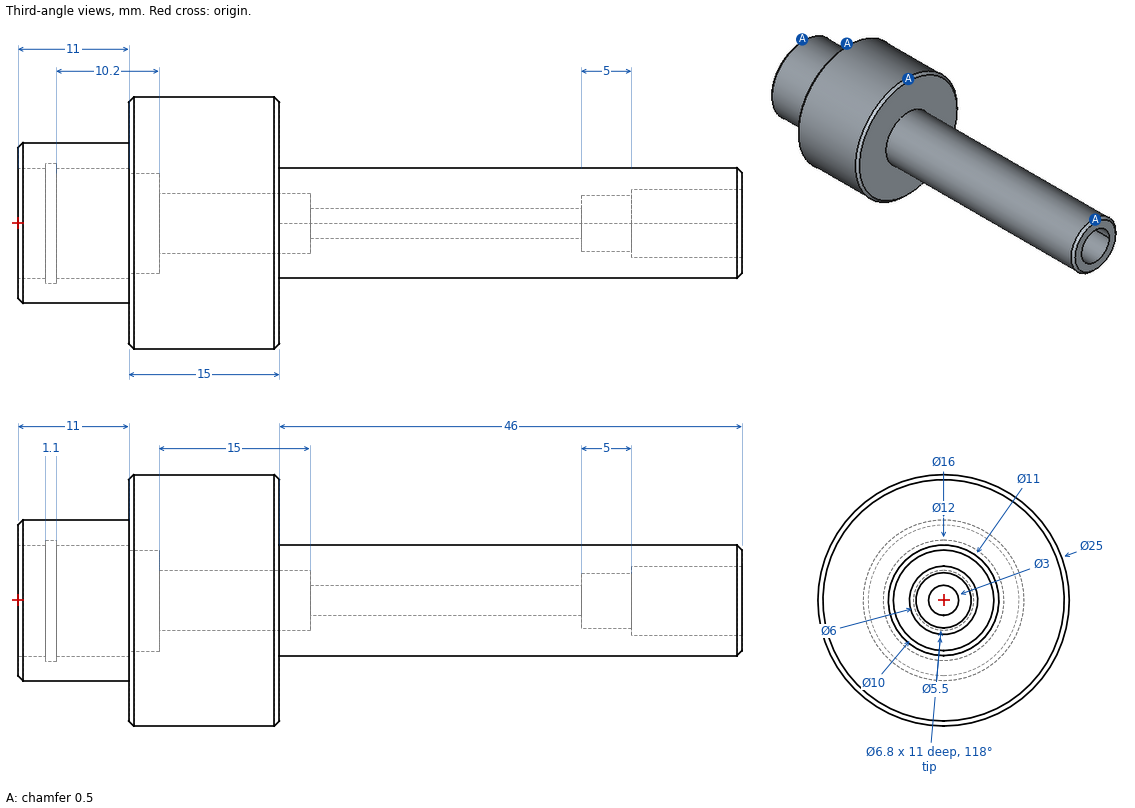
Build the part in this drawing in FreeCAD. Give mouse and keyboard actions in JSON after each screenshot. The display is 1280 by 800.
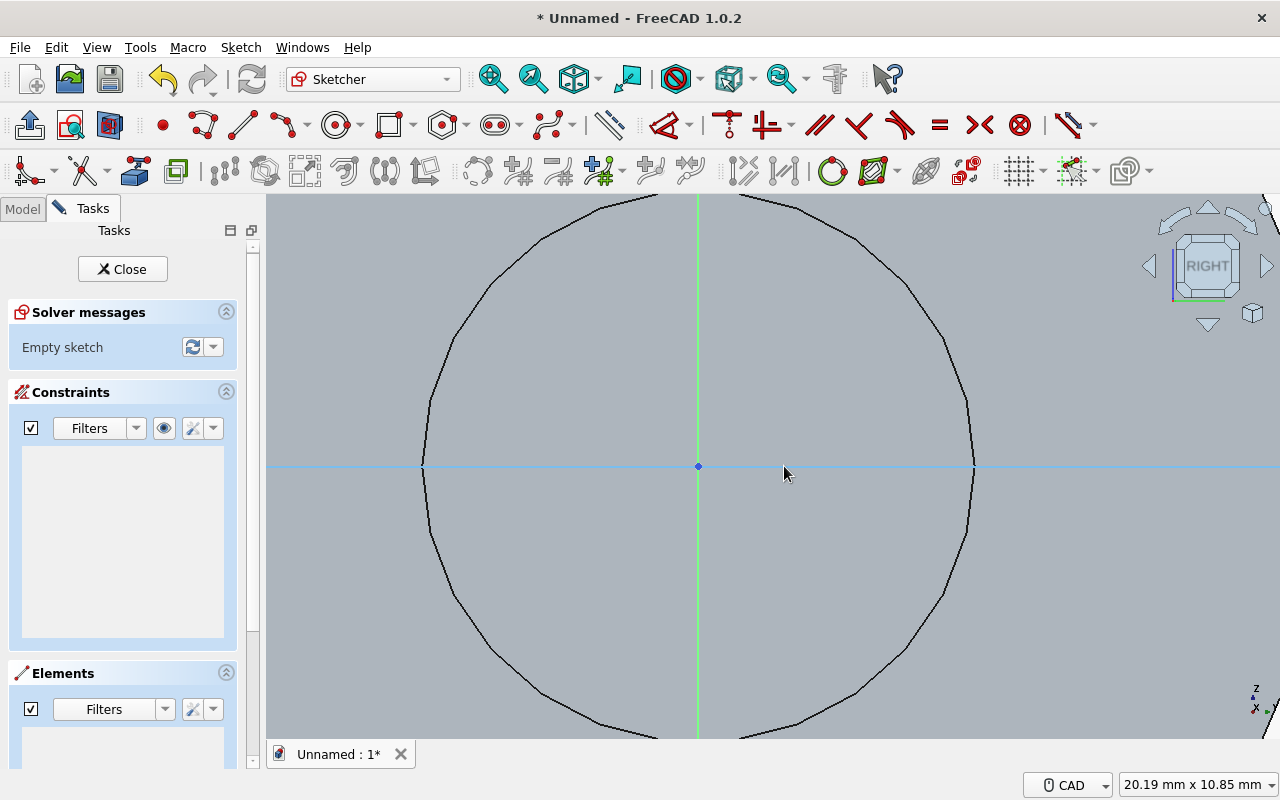
{"action": "left_click", "coordinate": [336, 126]}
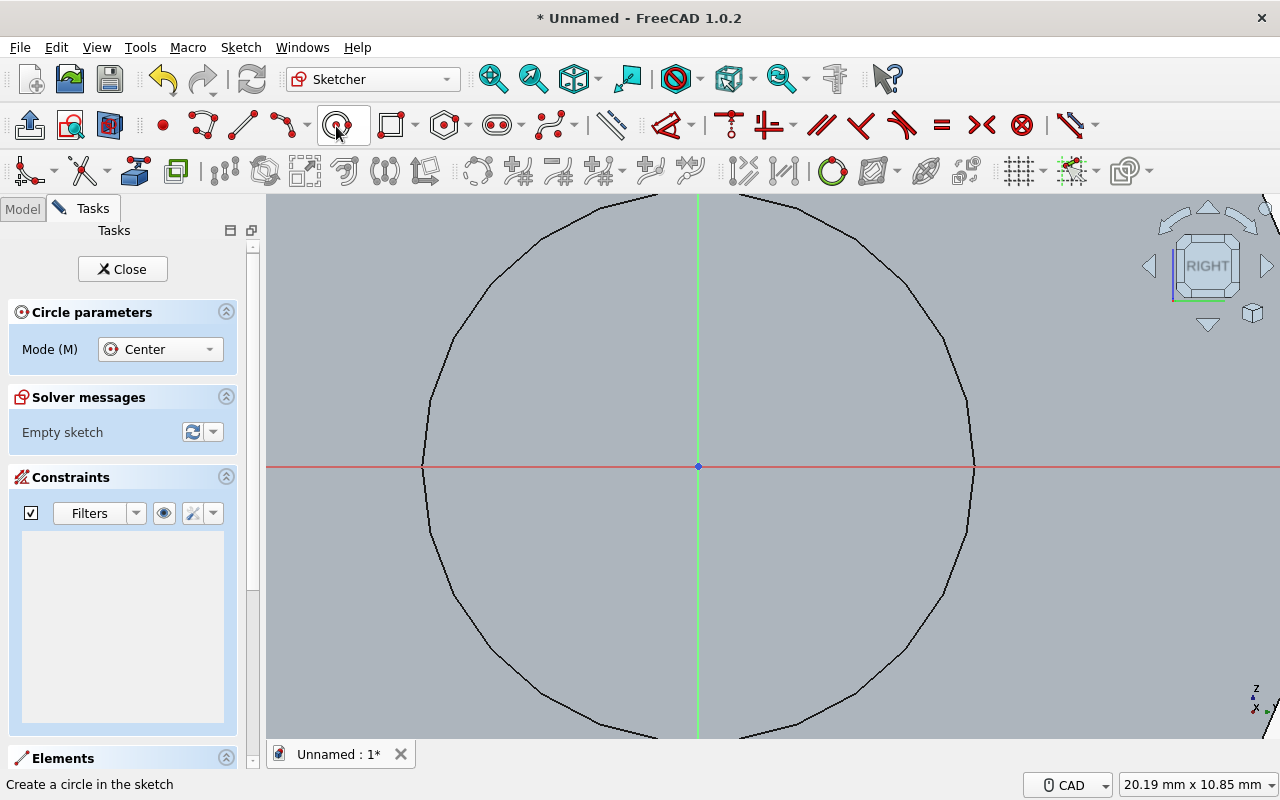
{"action": "left_click", "coordinate": [698, 466]}
{"action": "mouse_move", "coordinate": [819, 346]}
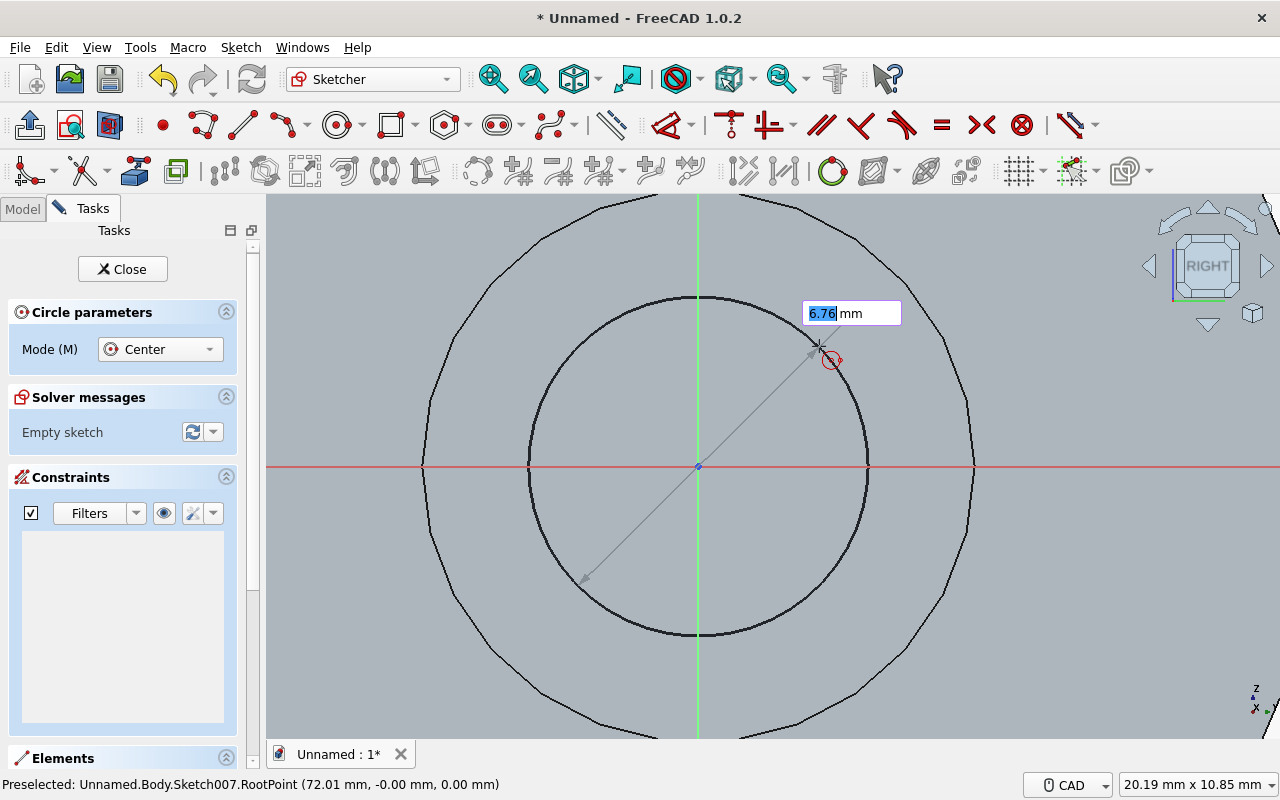
{"action": "type", "text": "6.8"}
{"action": "key", "text": "Return"}
{"action": "key", "text": "Escape"}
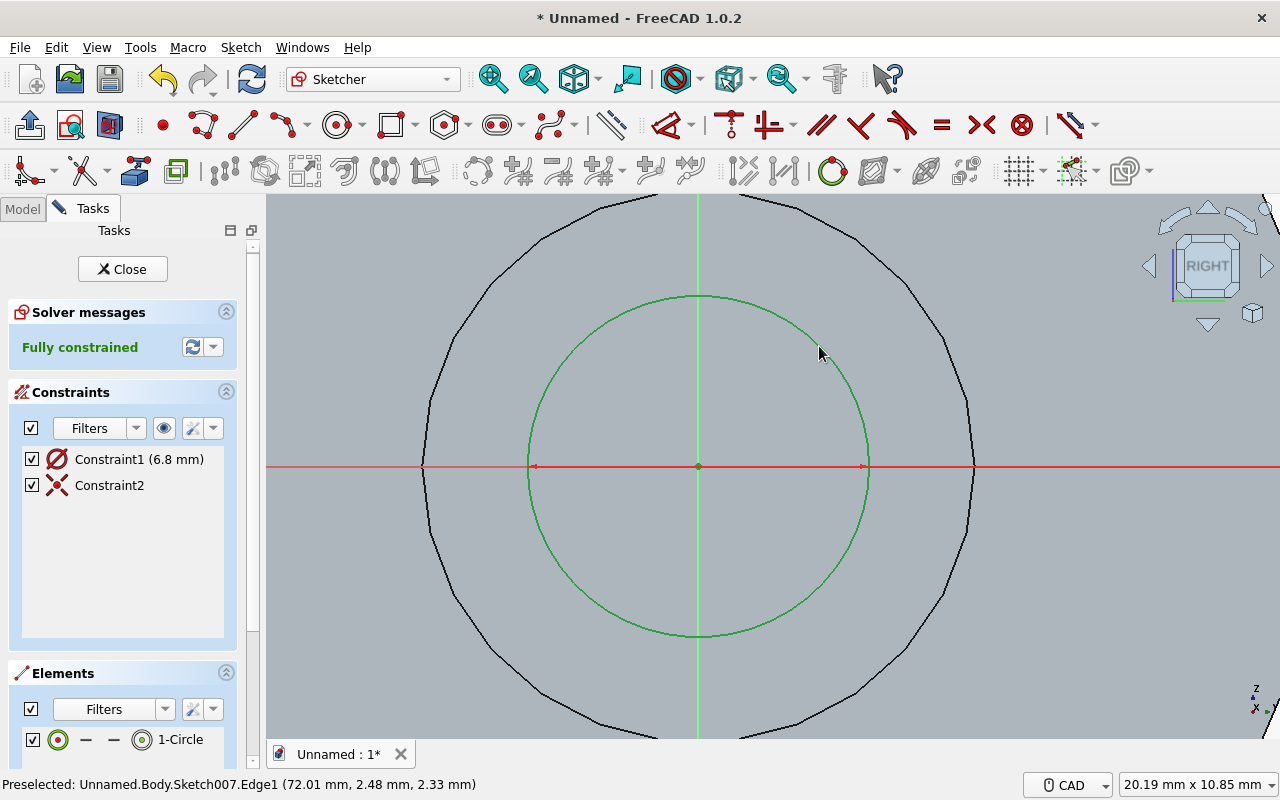
{"action": "left_click", "coordinate": [123, 269]}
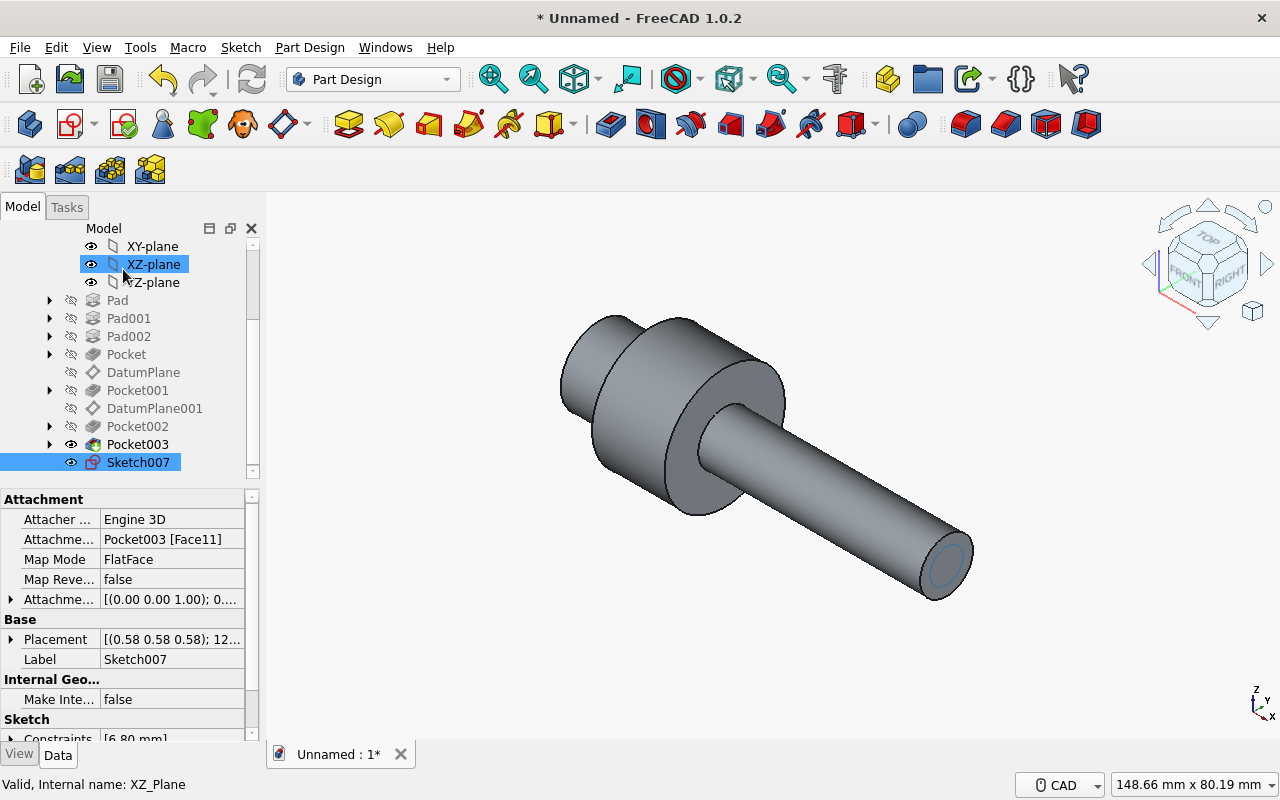
{"action": "left_click", "coordinate": [652, 124]}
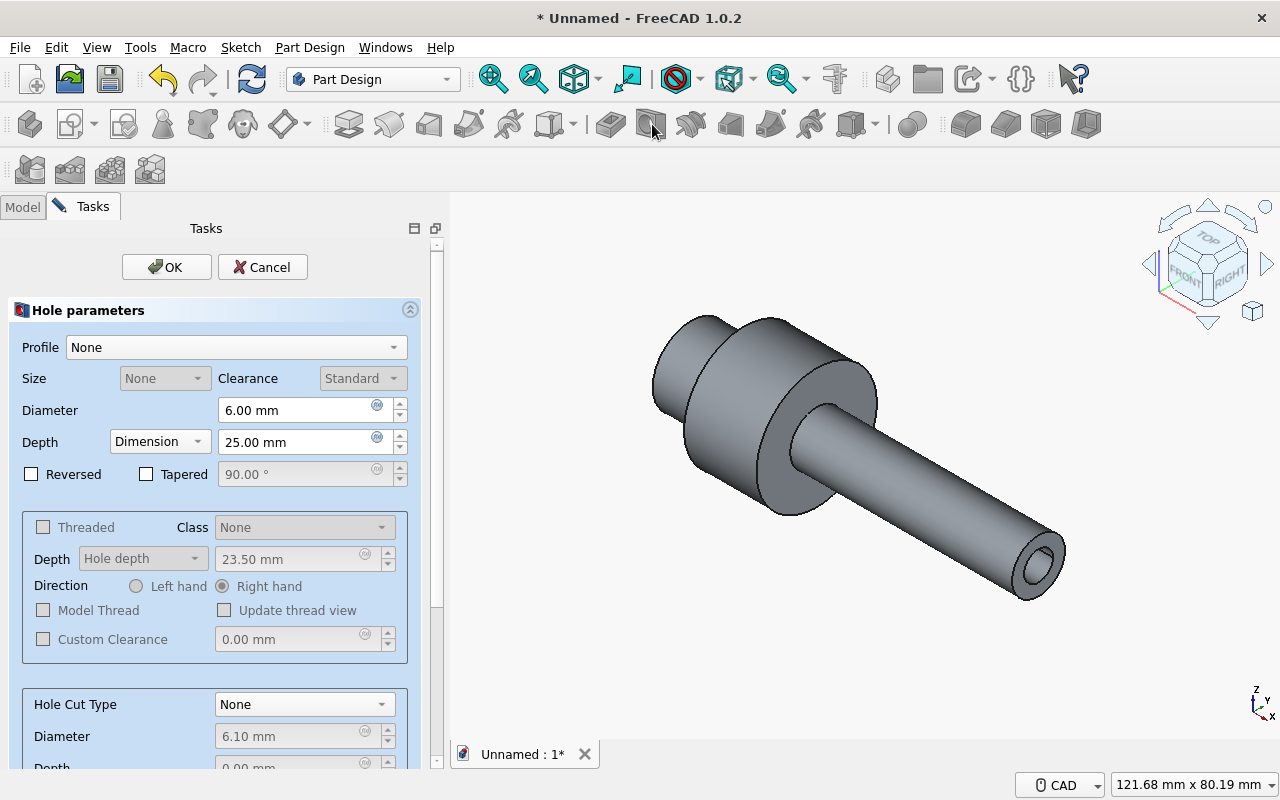
{"action": "triple_click", "coordinate": [305, 410]}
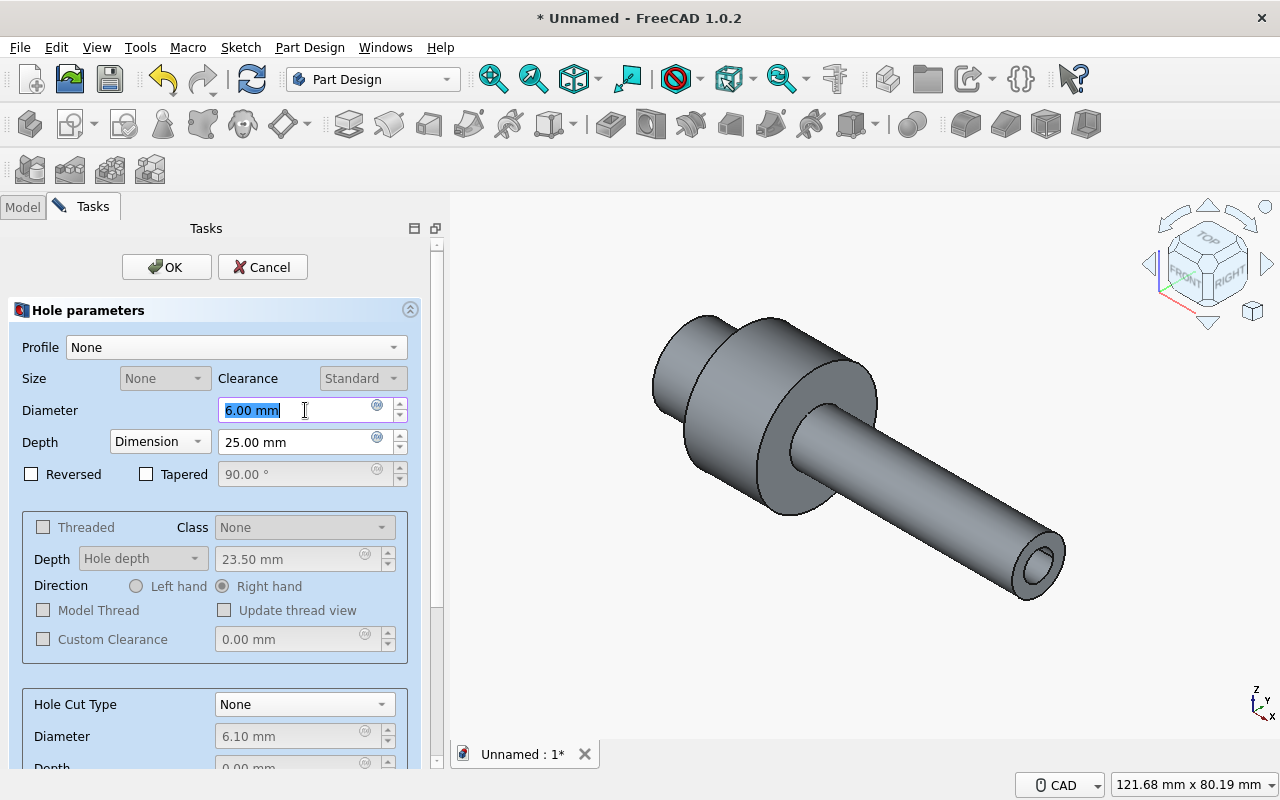
{"action": "type", "text": "6.8"}
{"action": "key", "text": "Tab"}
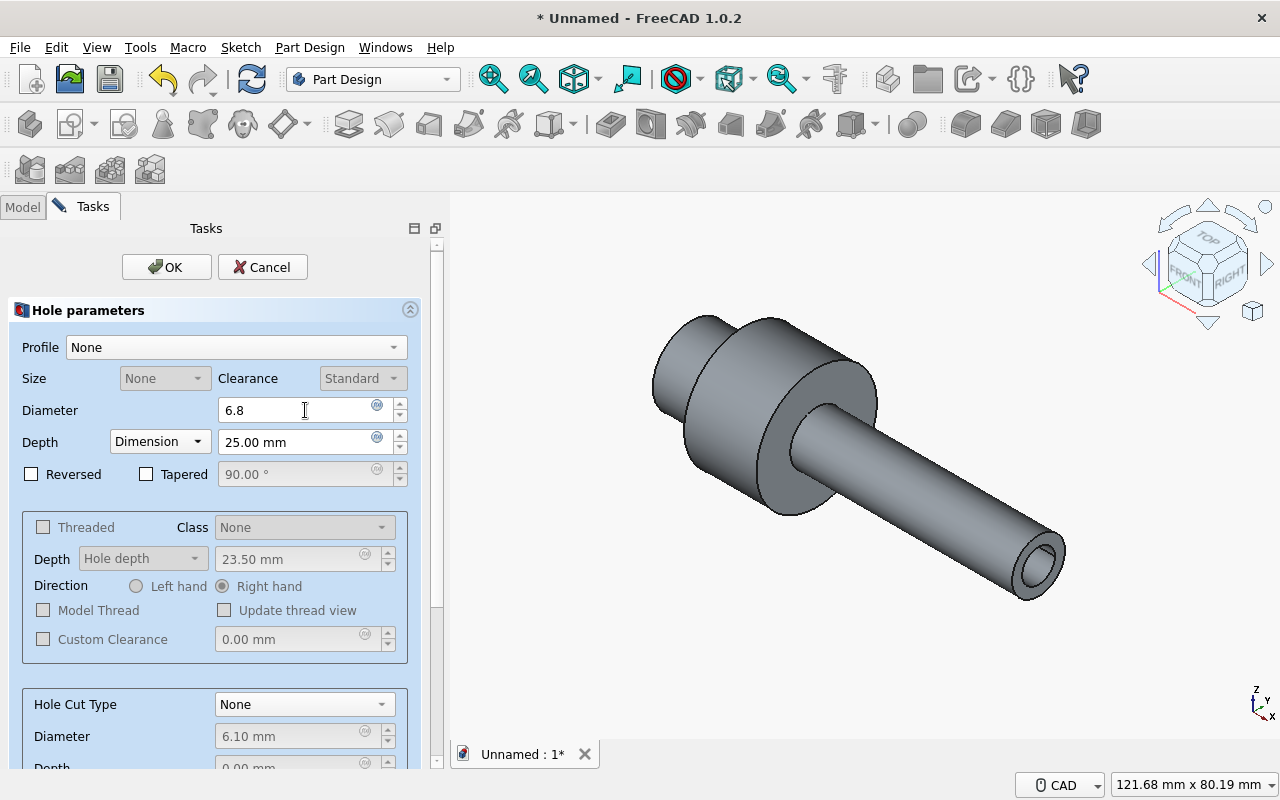
{"action": "triple_click", "coordinate": [305, 442]}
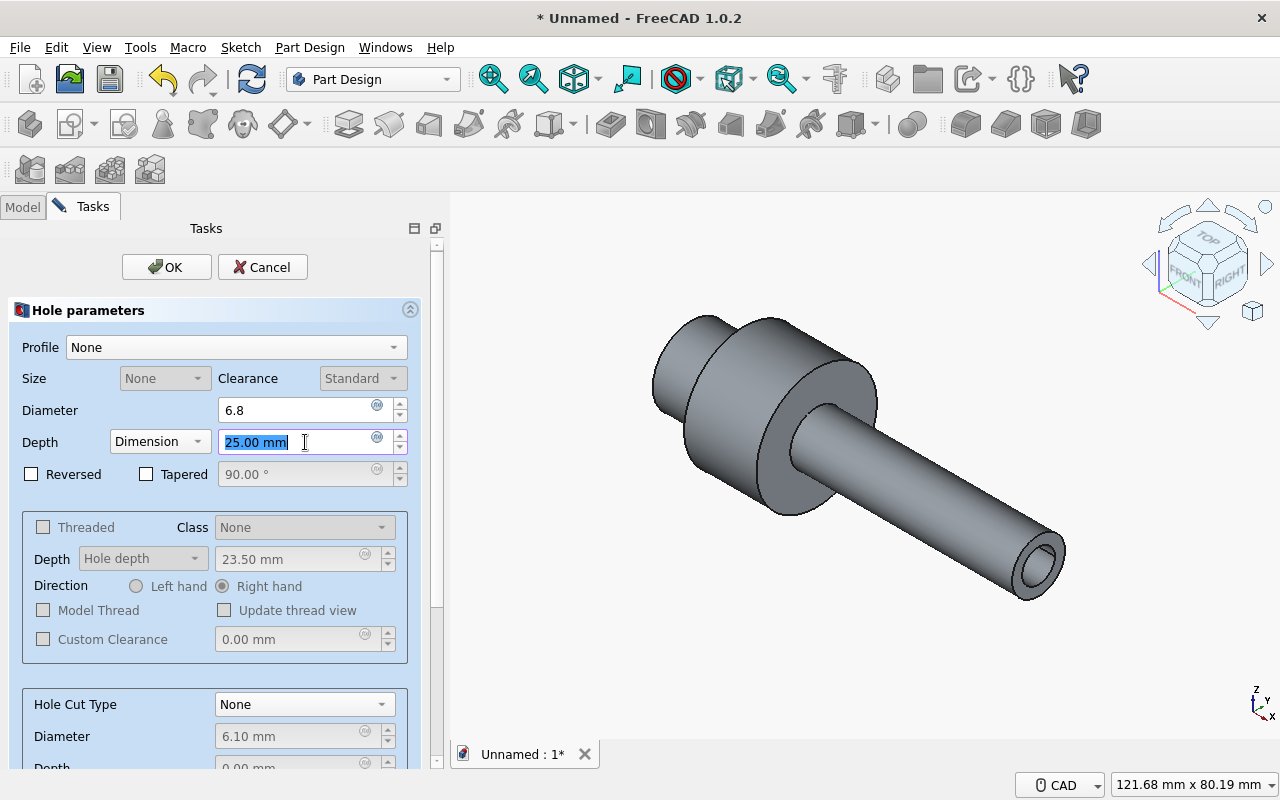
{"action": "type", "text": "11"}
{"action": "key", "text": "Tab"}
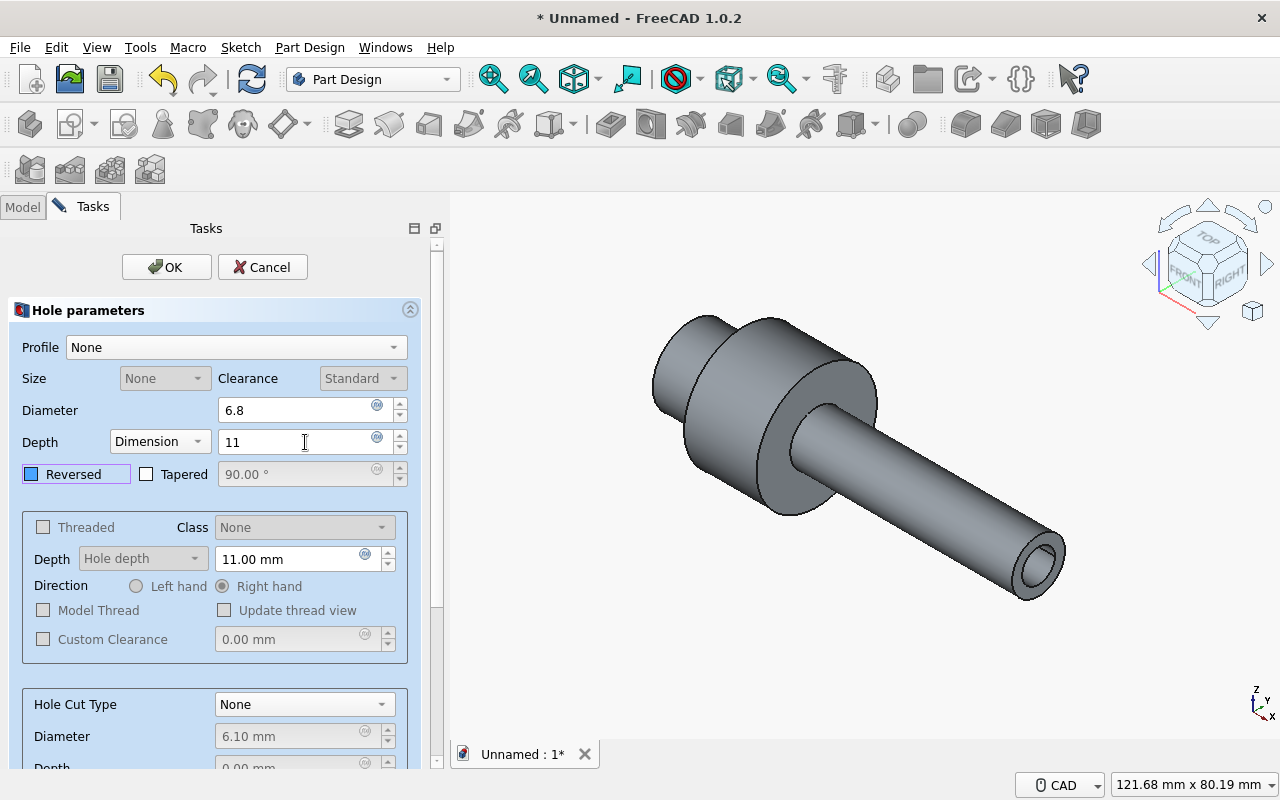
{"action": "left_click", "coordinate": [167, 267]}